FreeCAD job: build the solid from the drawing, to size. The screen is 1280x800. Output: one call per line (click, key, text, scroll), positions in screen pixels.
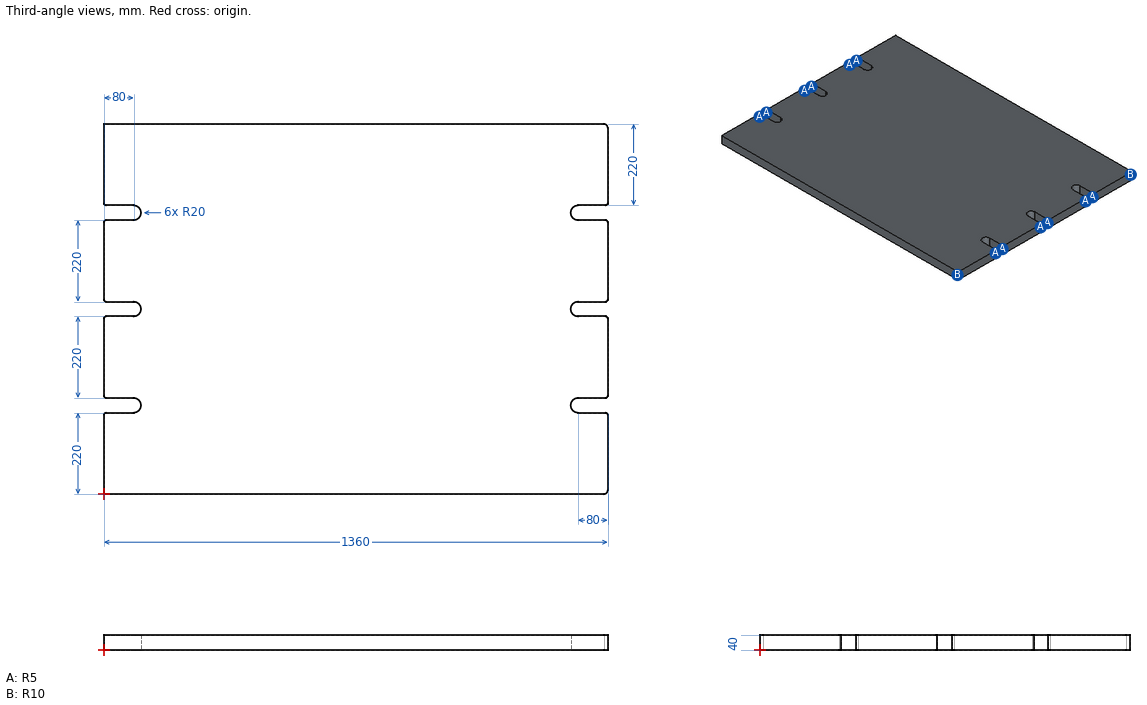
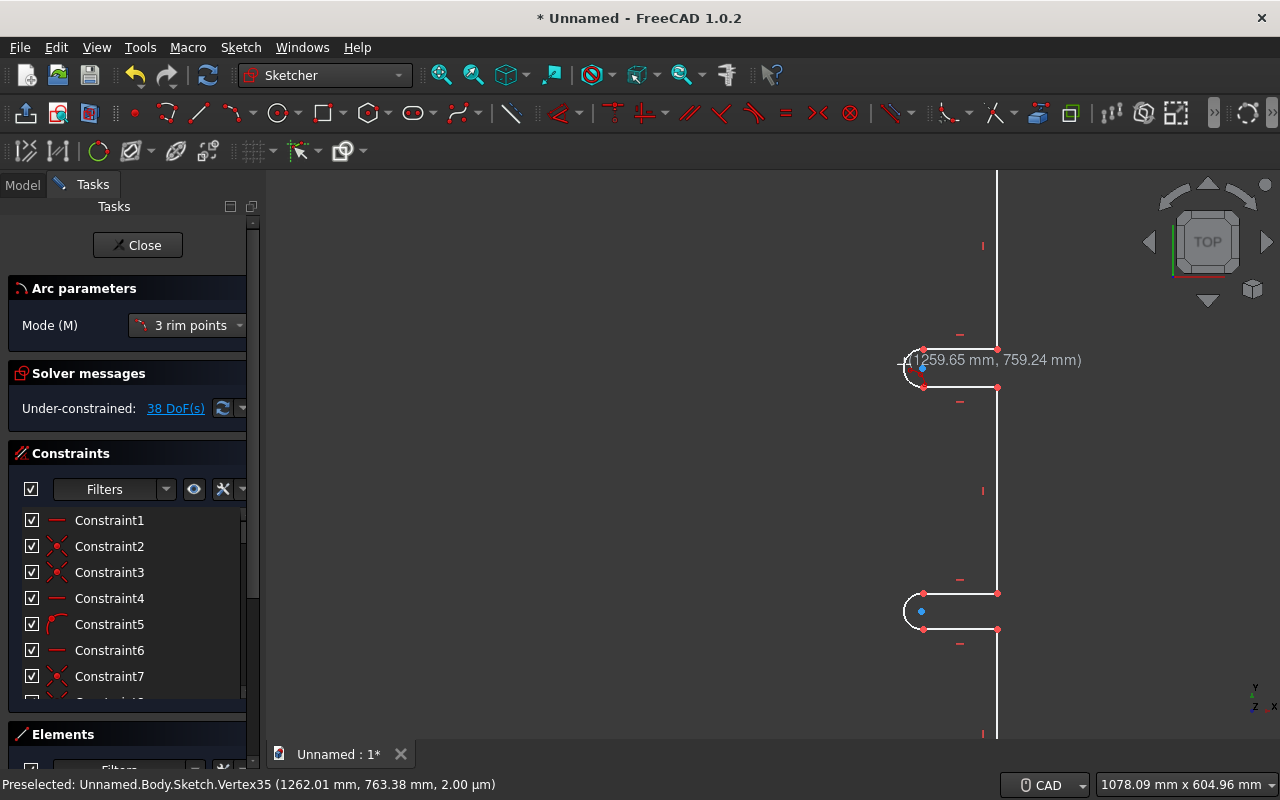
scroll(906, 365, down, 5)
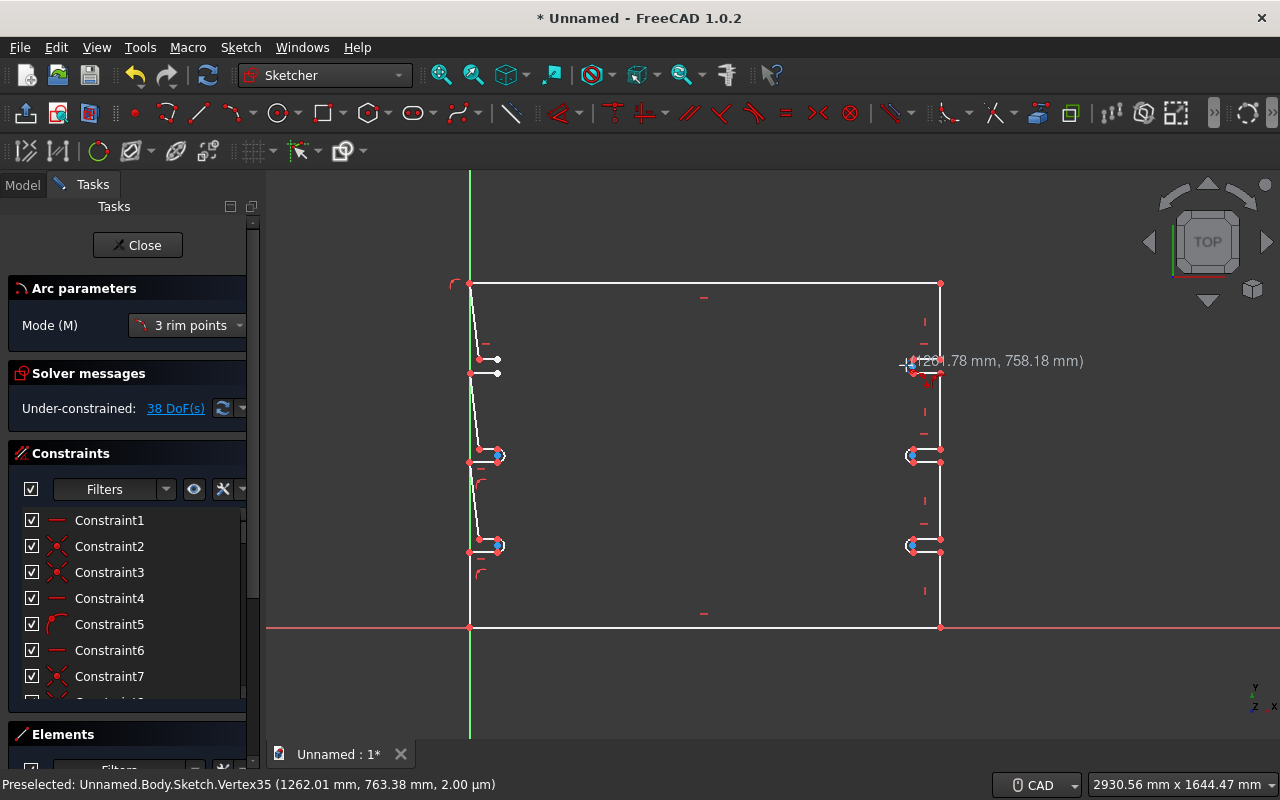
click(497, 359)
click(497, 373)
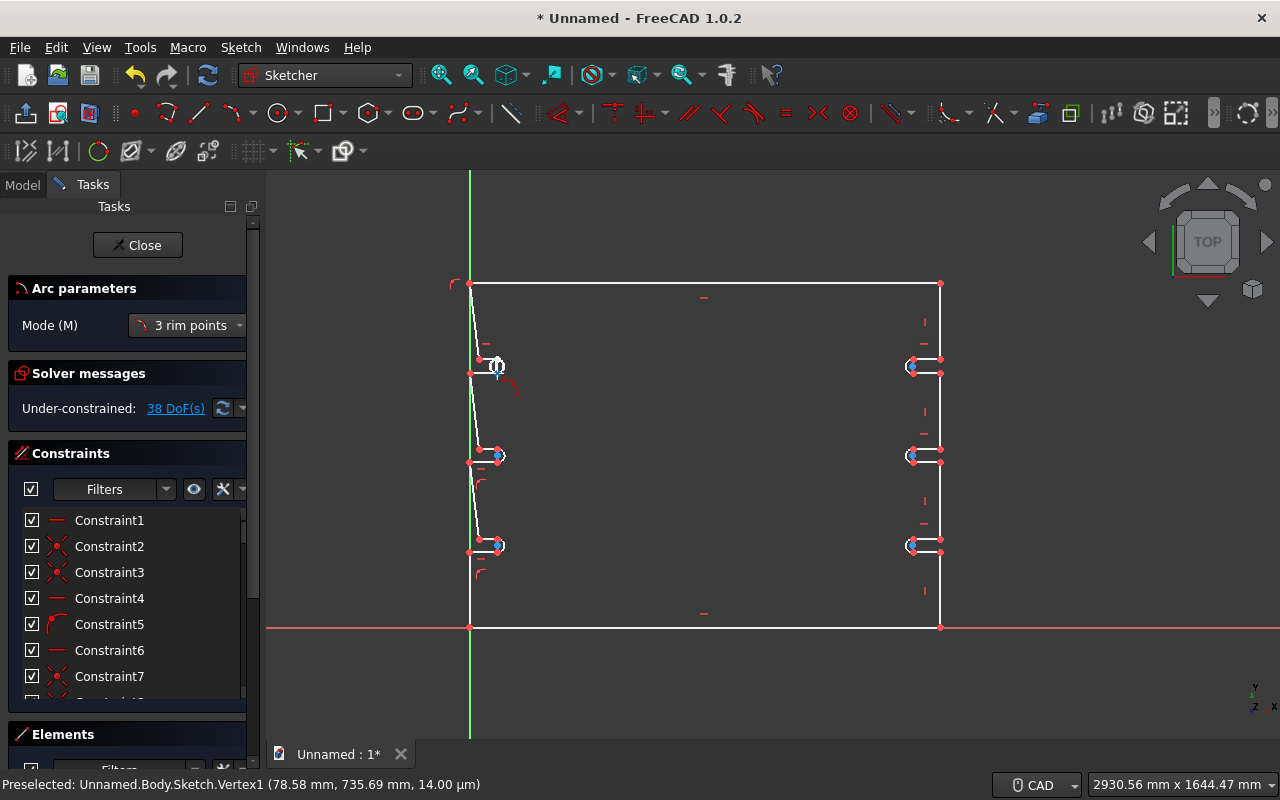
scroll(504, 365, up, 5)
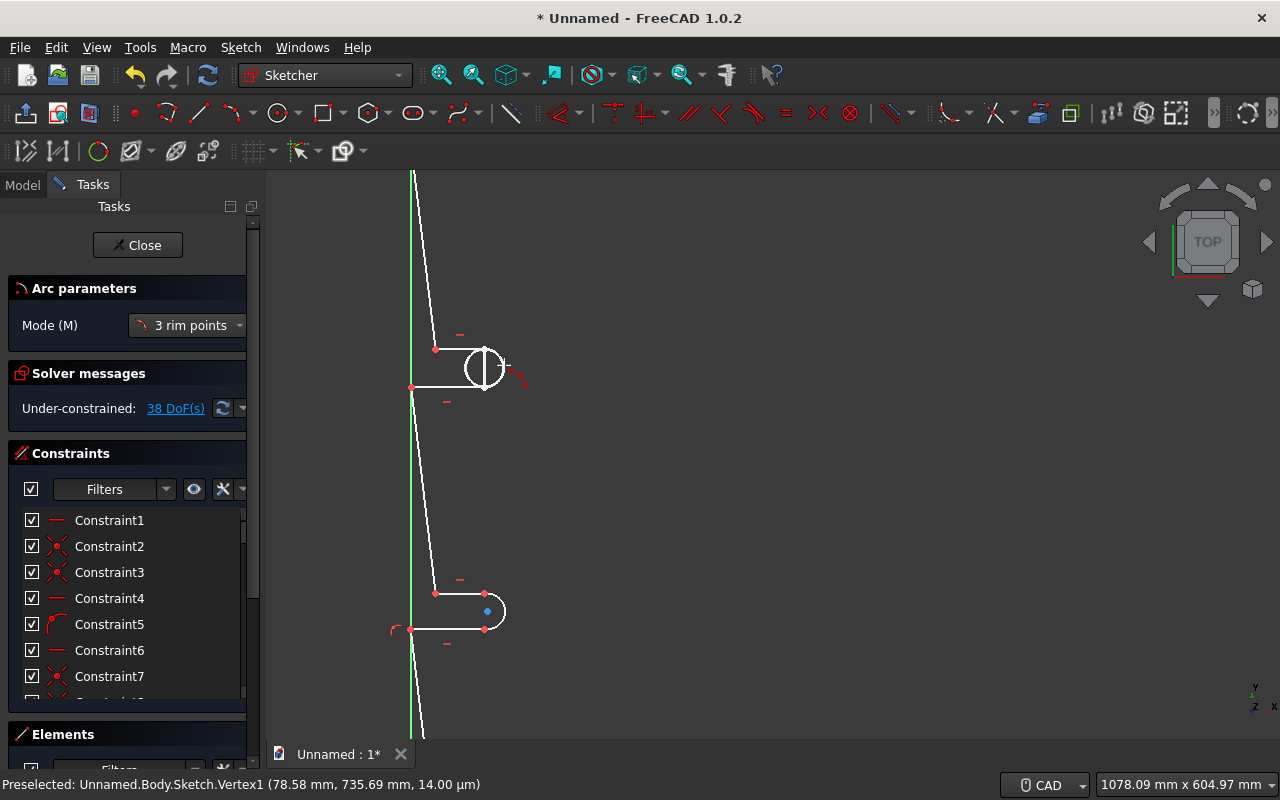
click(505, 364)
key(Escape)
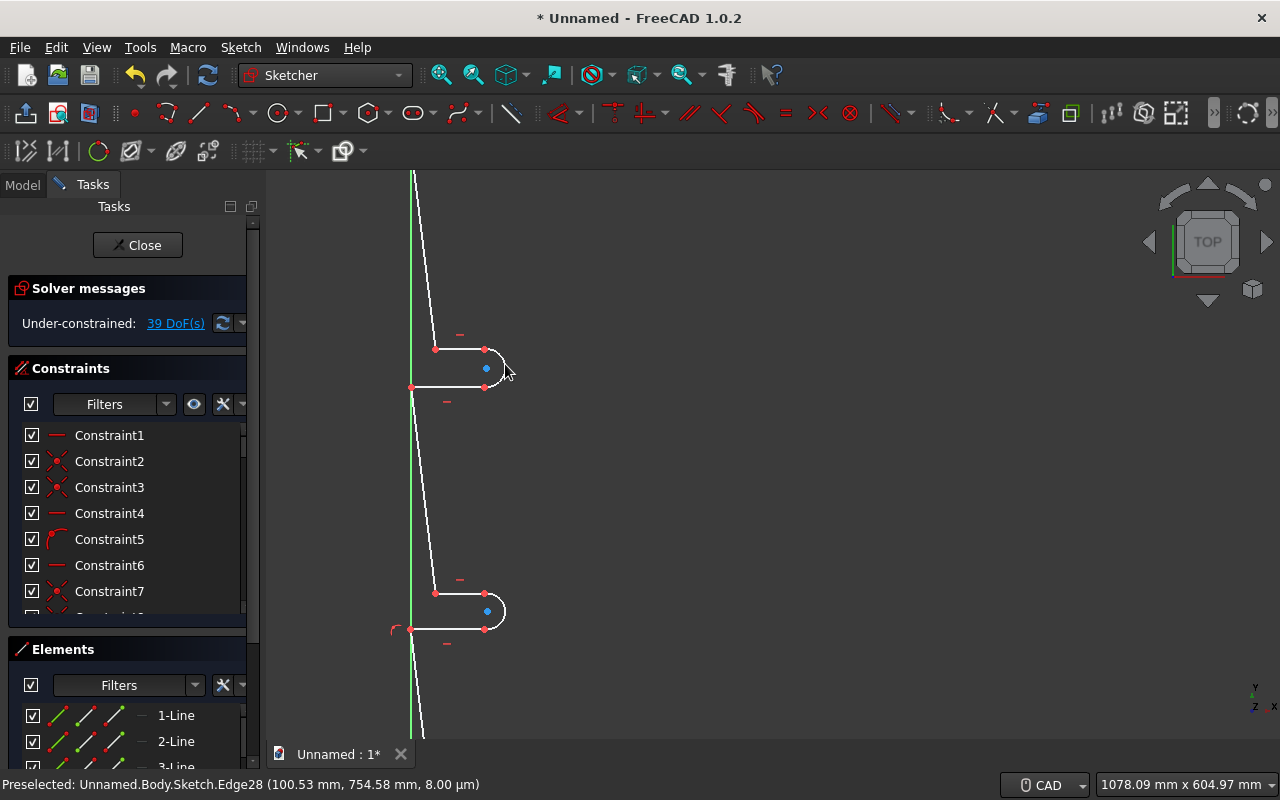
click(463, 387)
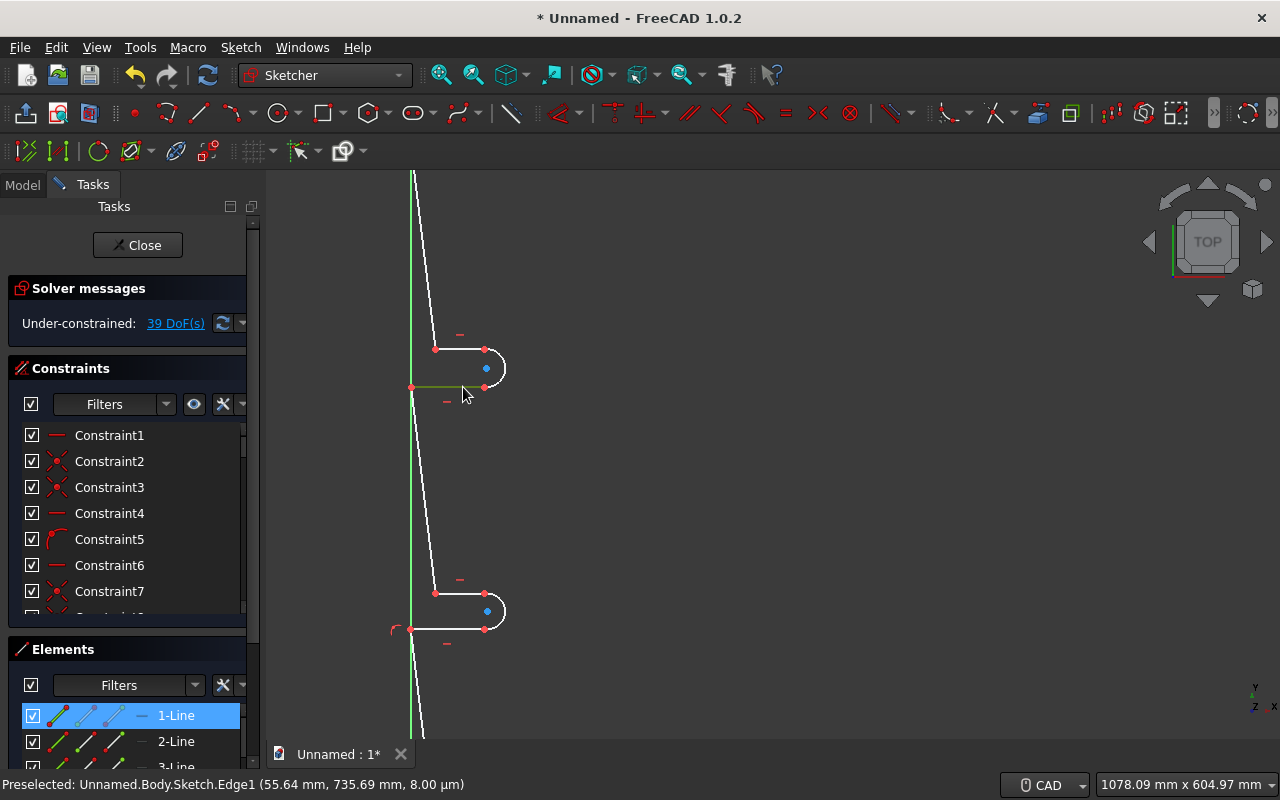
click(501, 380)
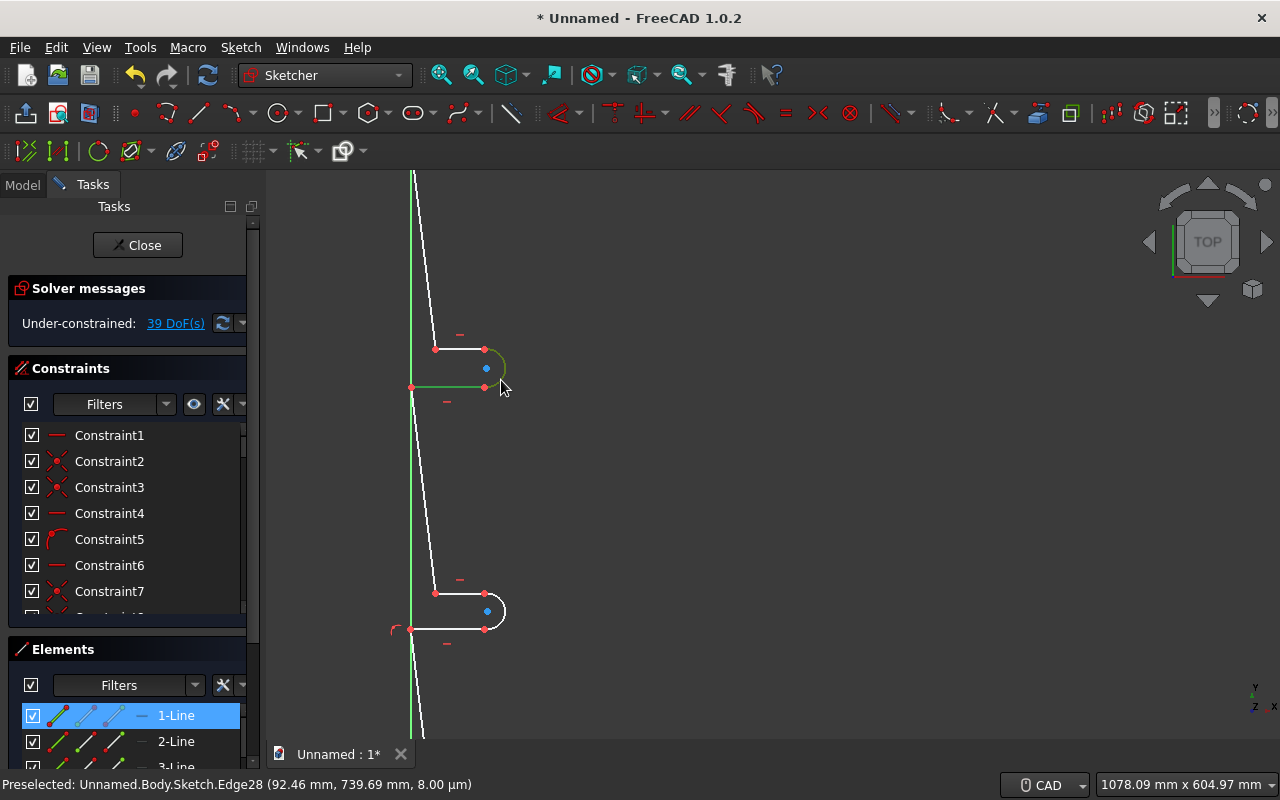
click(754, 114)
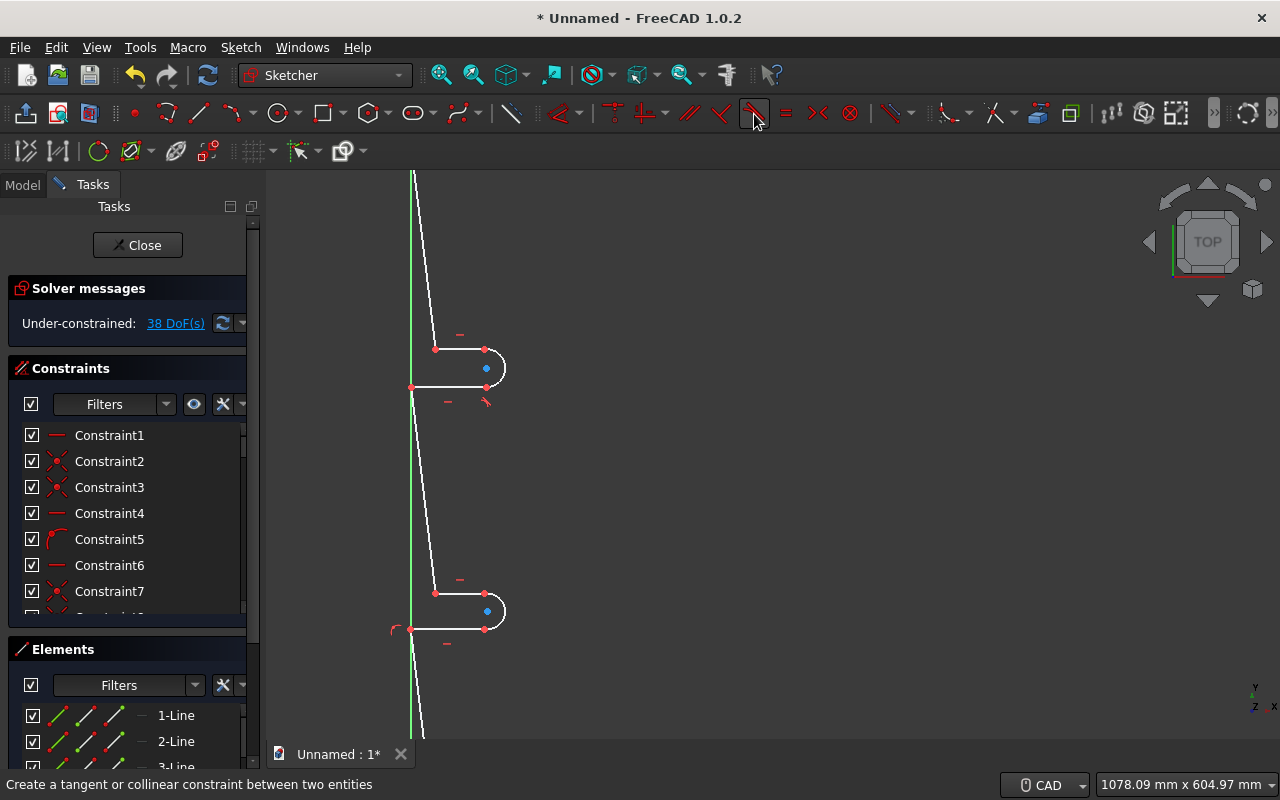
click(450, 594)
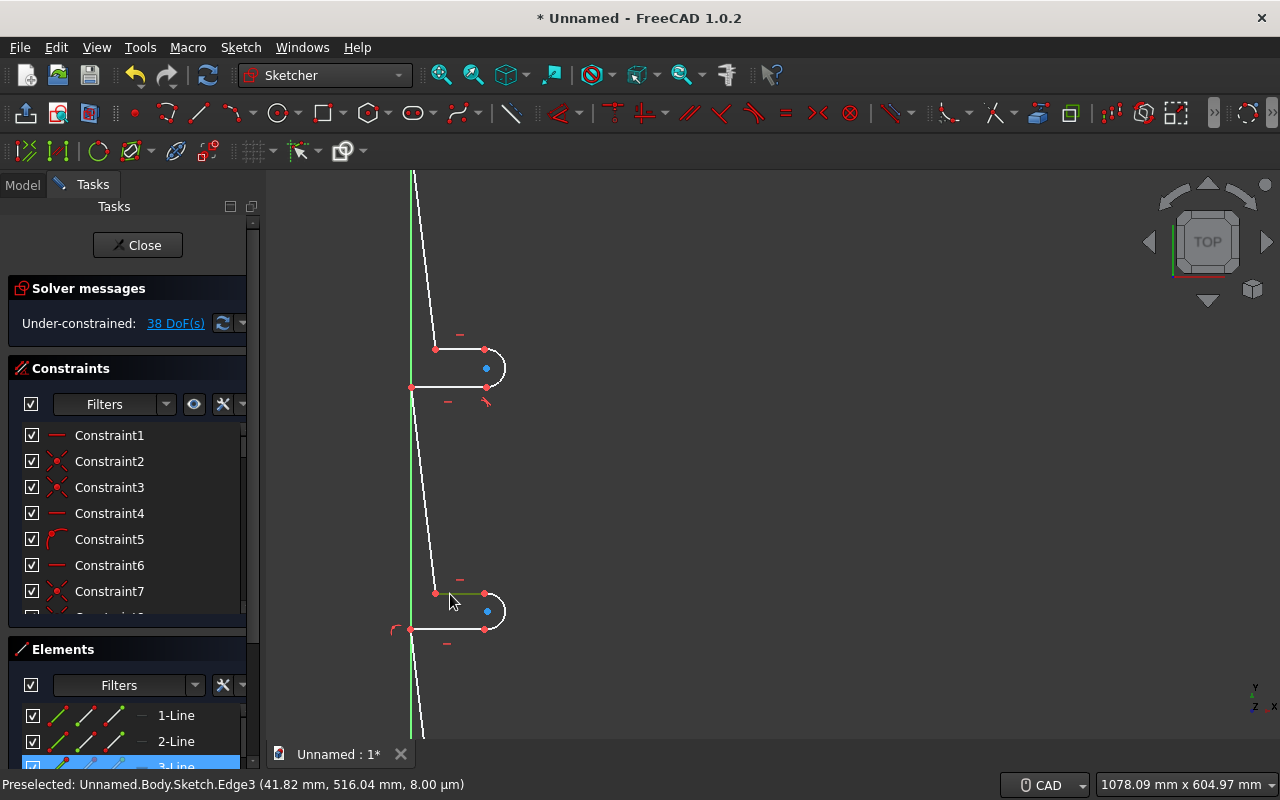
click(501, 623)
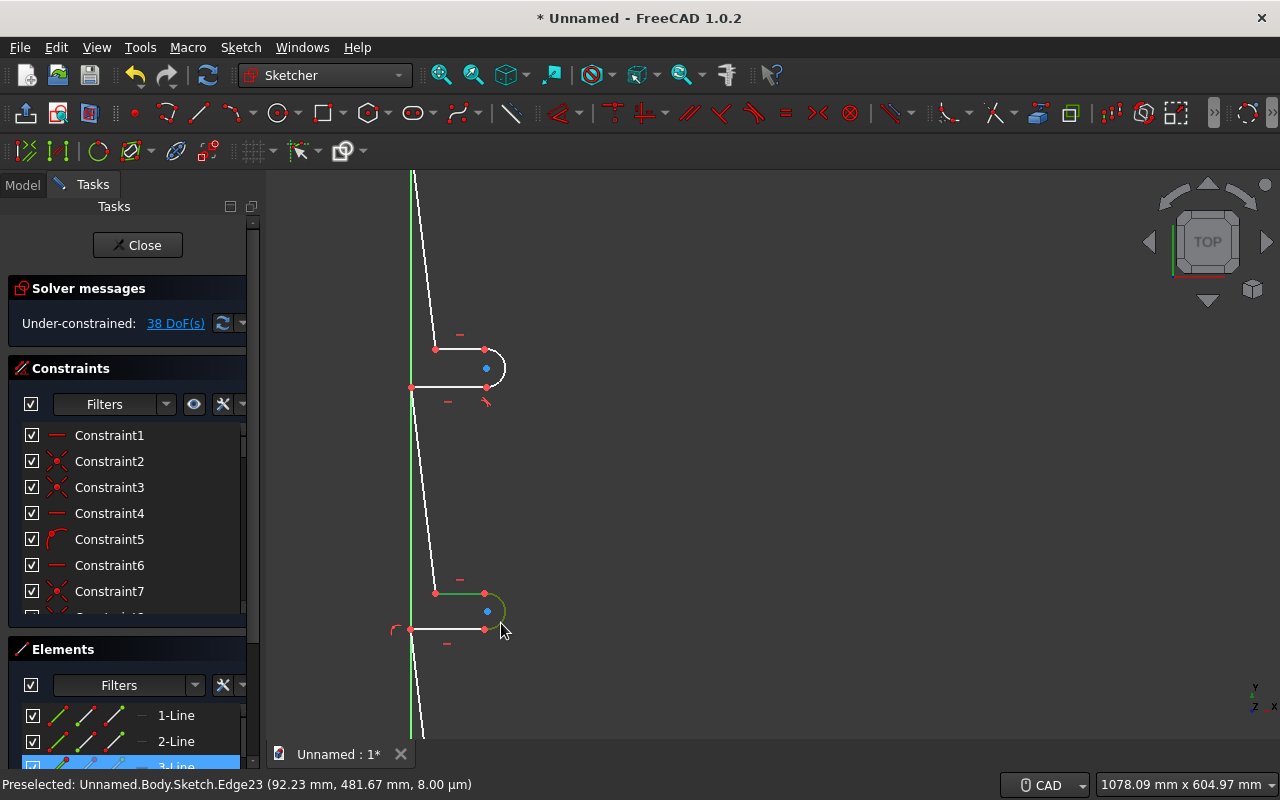
click(754, 114)